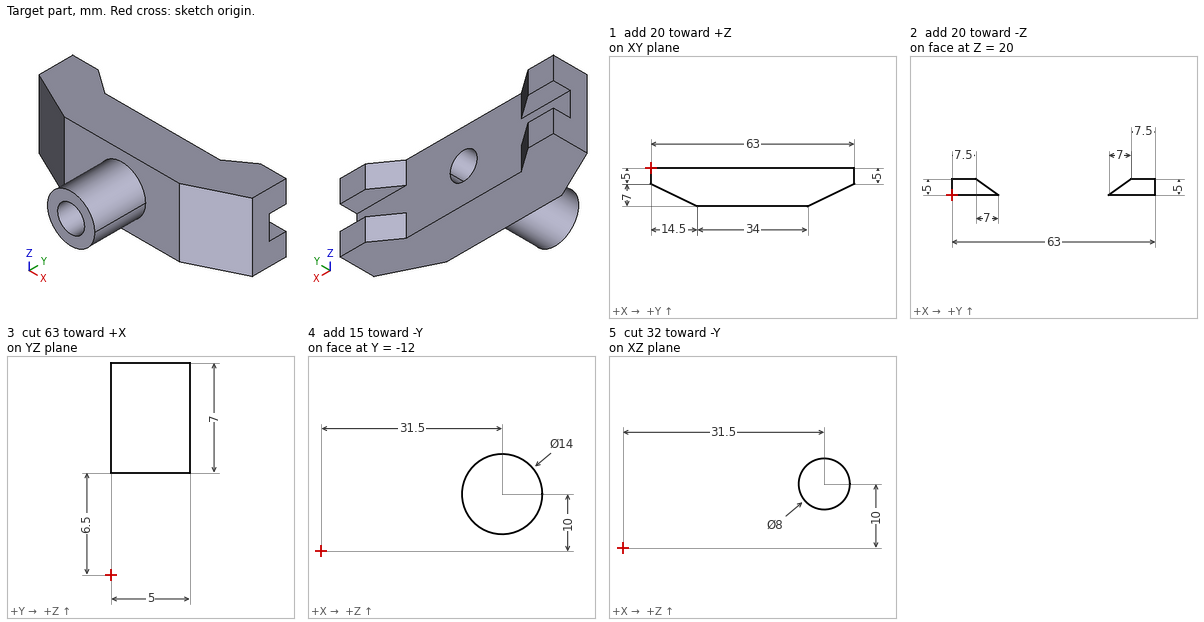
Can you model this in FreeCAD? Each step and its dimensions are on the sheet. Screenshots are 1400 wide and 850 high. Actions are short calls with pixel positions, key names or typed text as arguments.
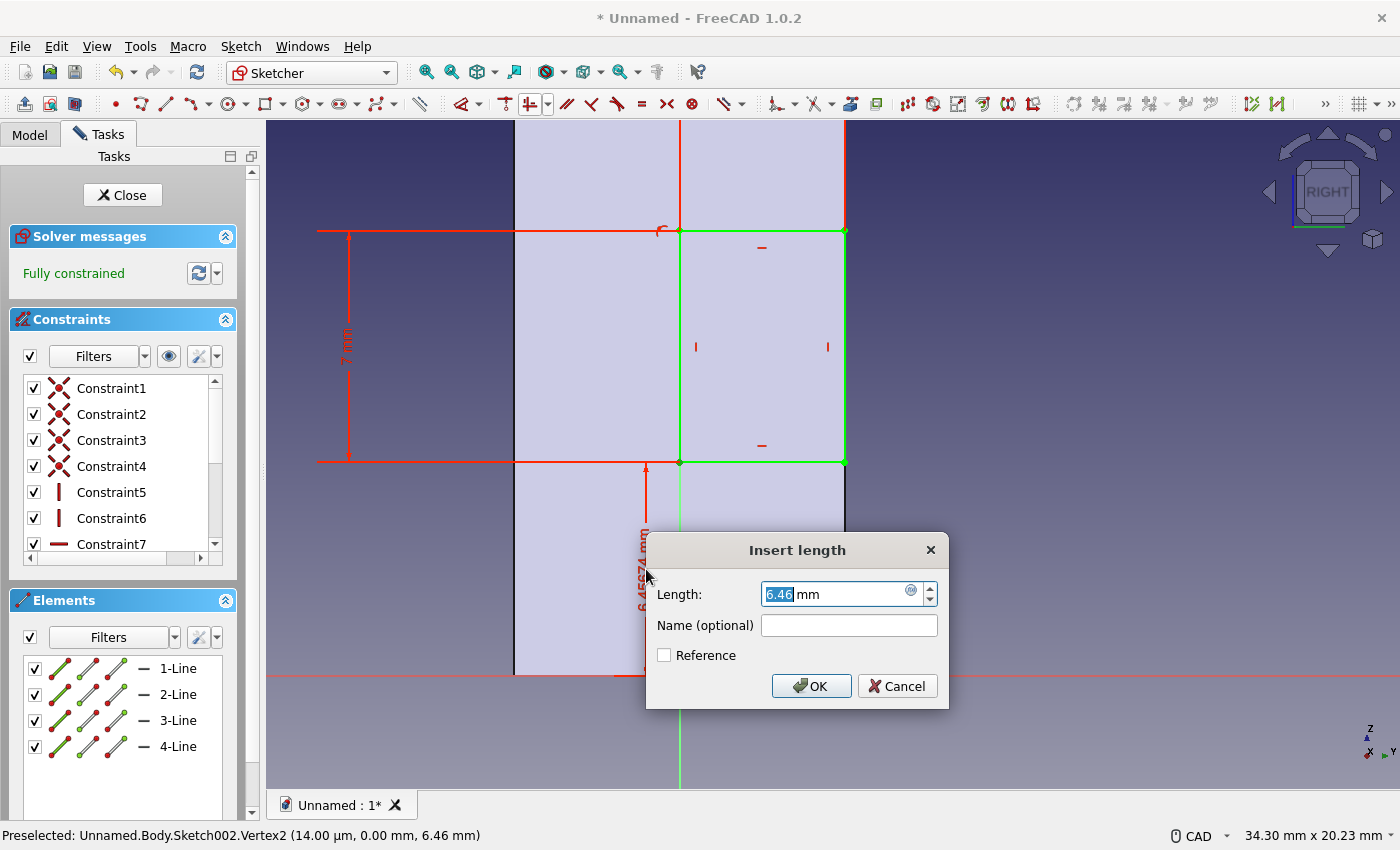
text(6.5)
key(Return)
key(Escape)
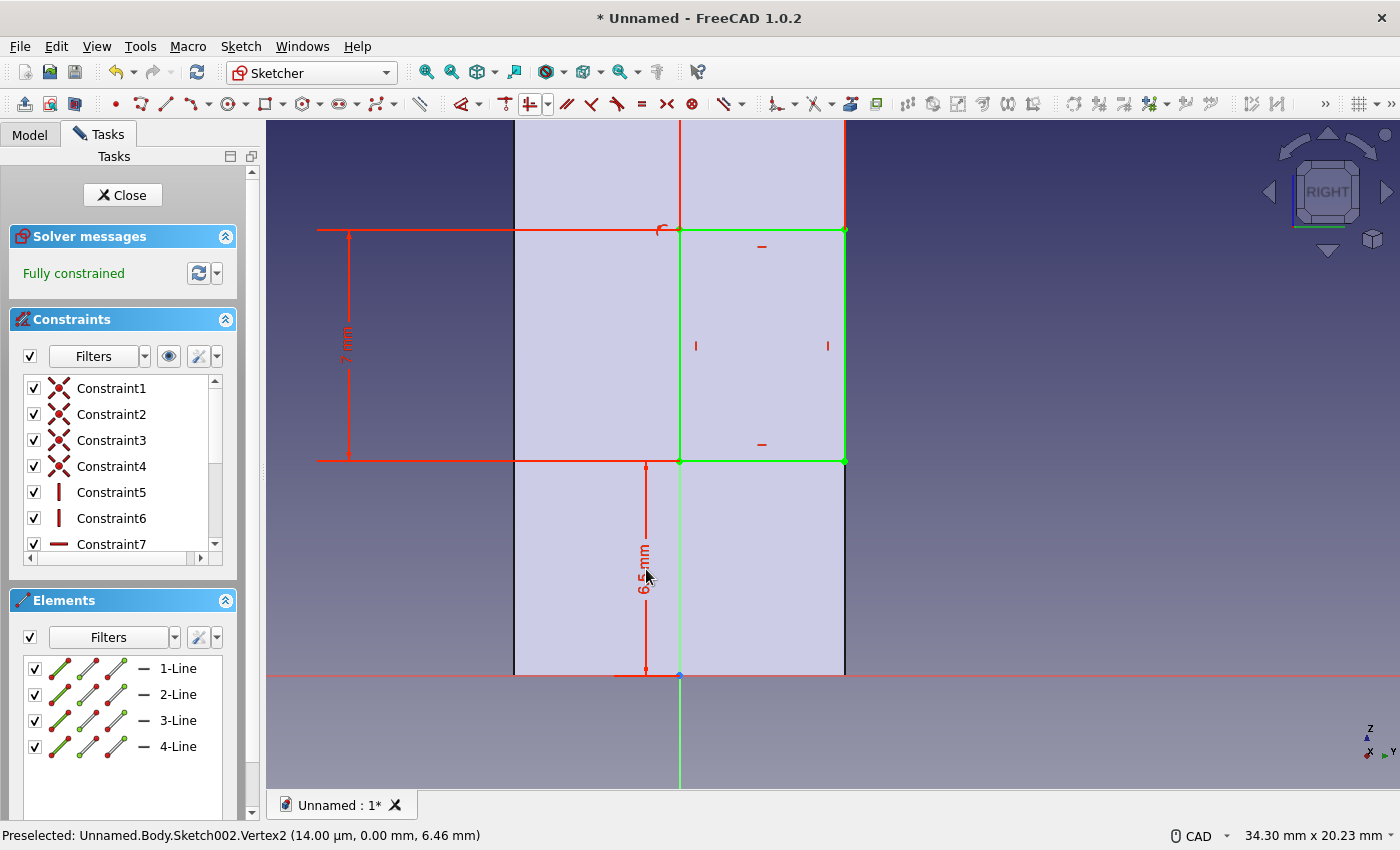
click(123, 195)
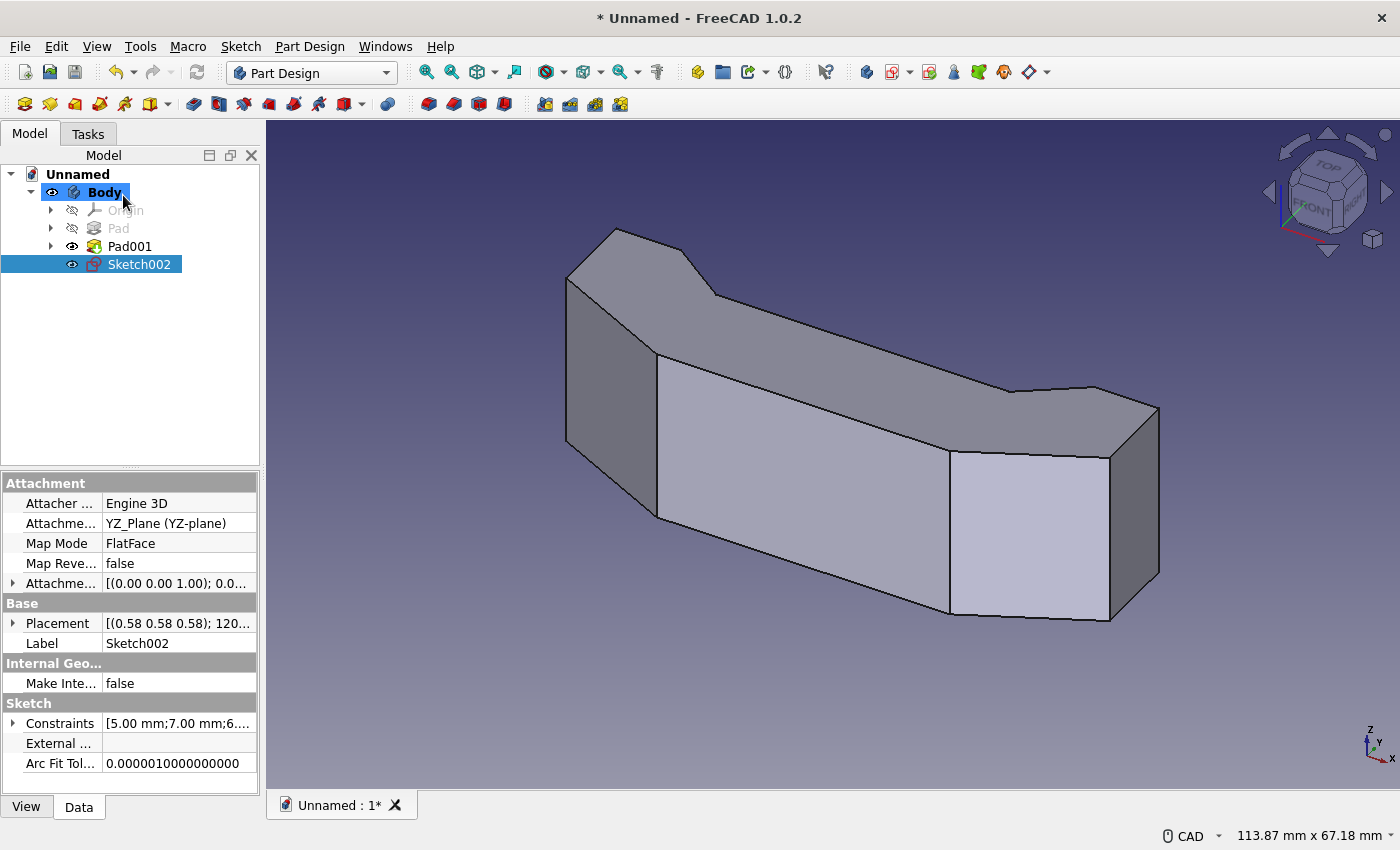
click(194, 104)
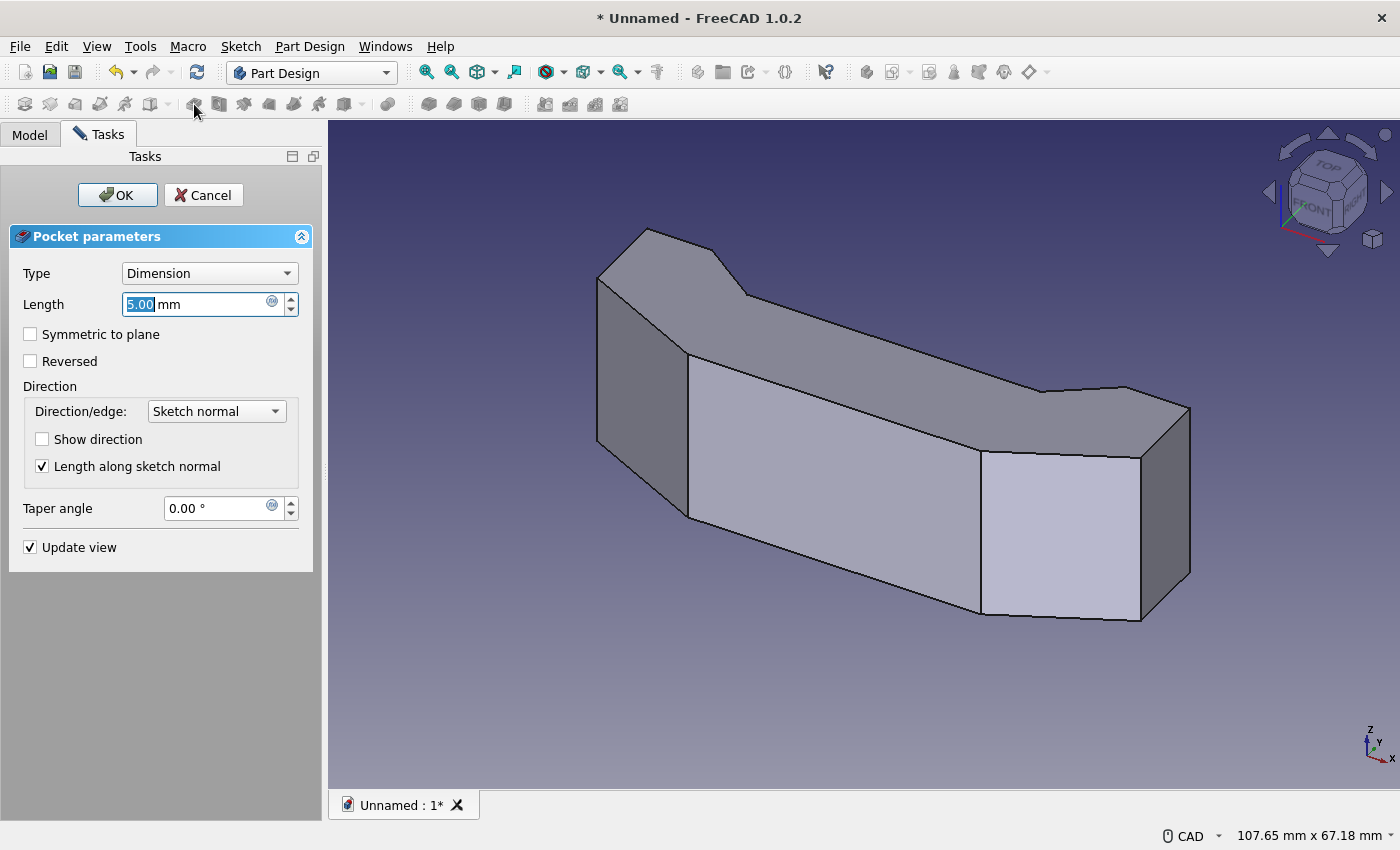
text(63)
key(Tab)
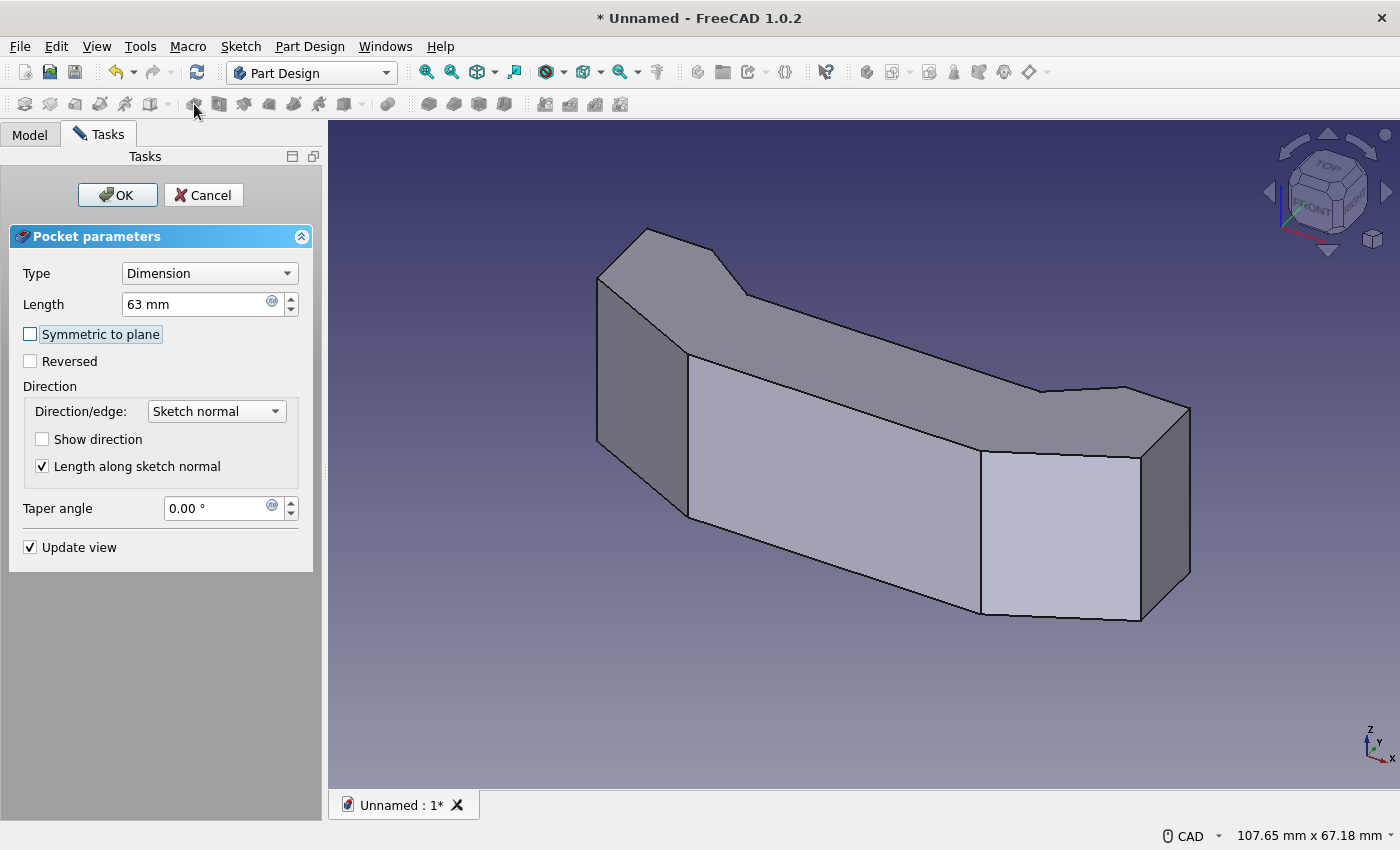
click(31, 361)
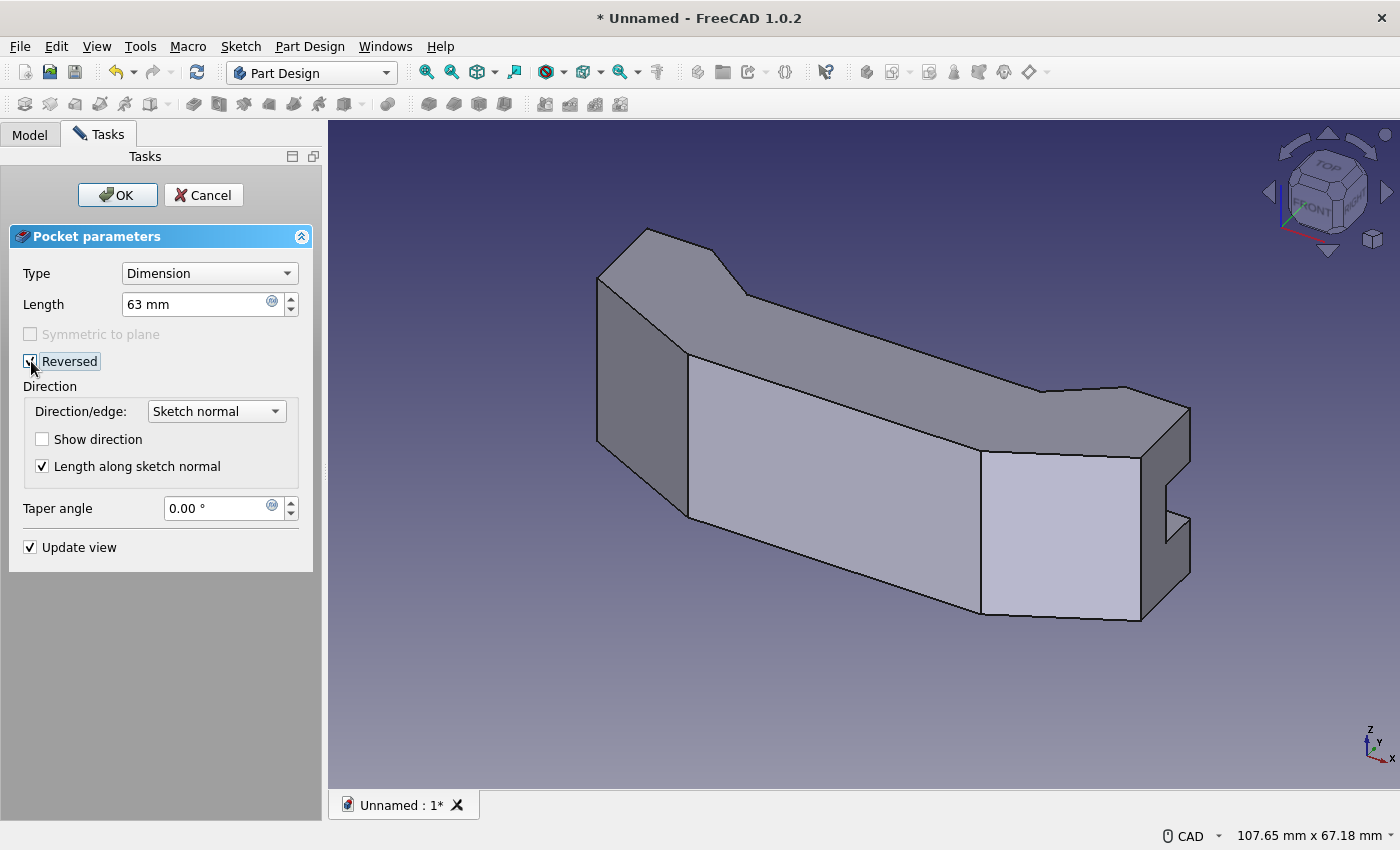
click(118, 195)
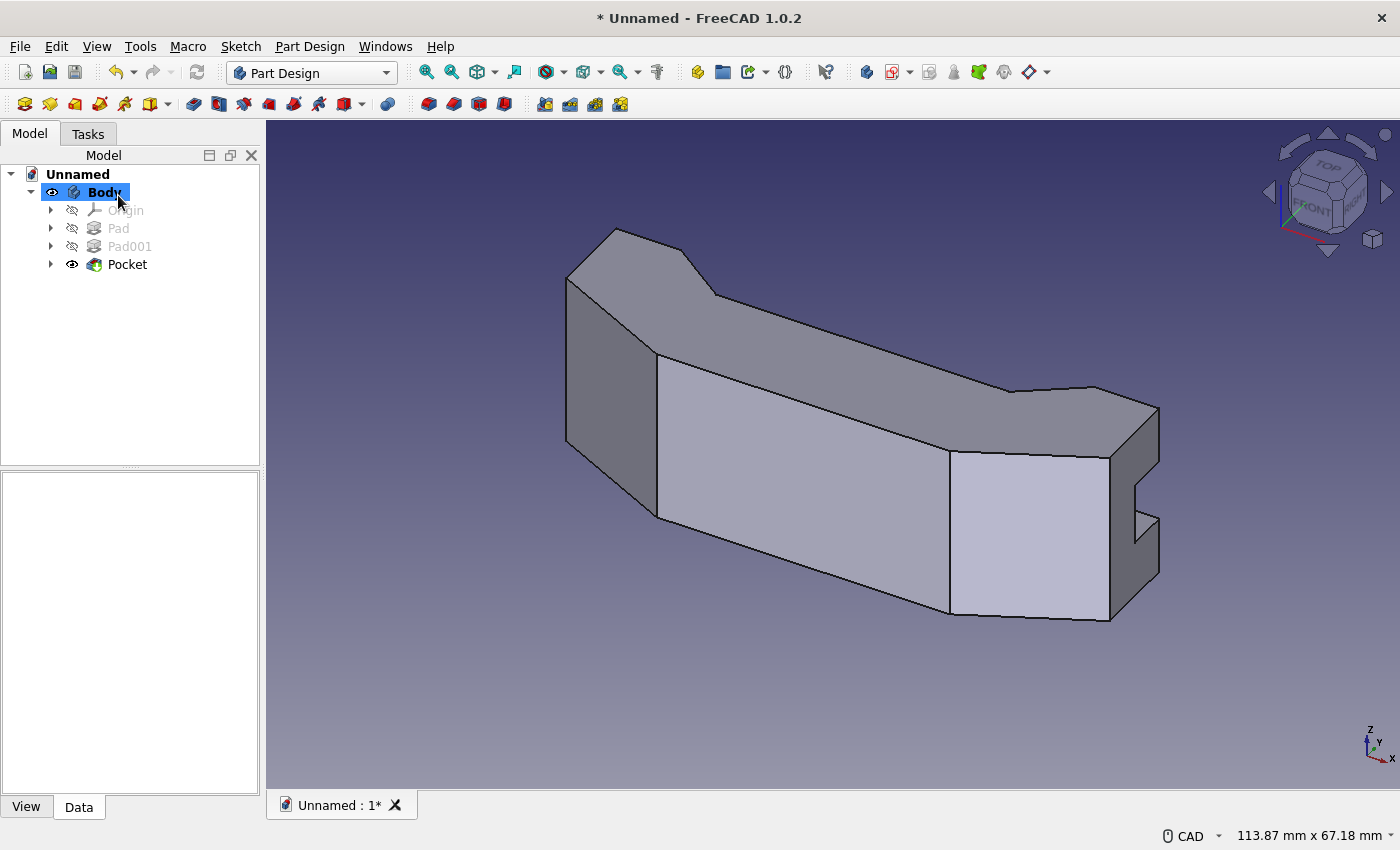
click(845, 497)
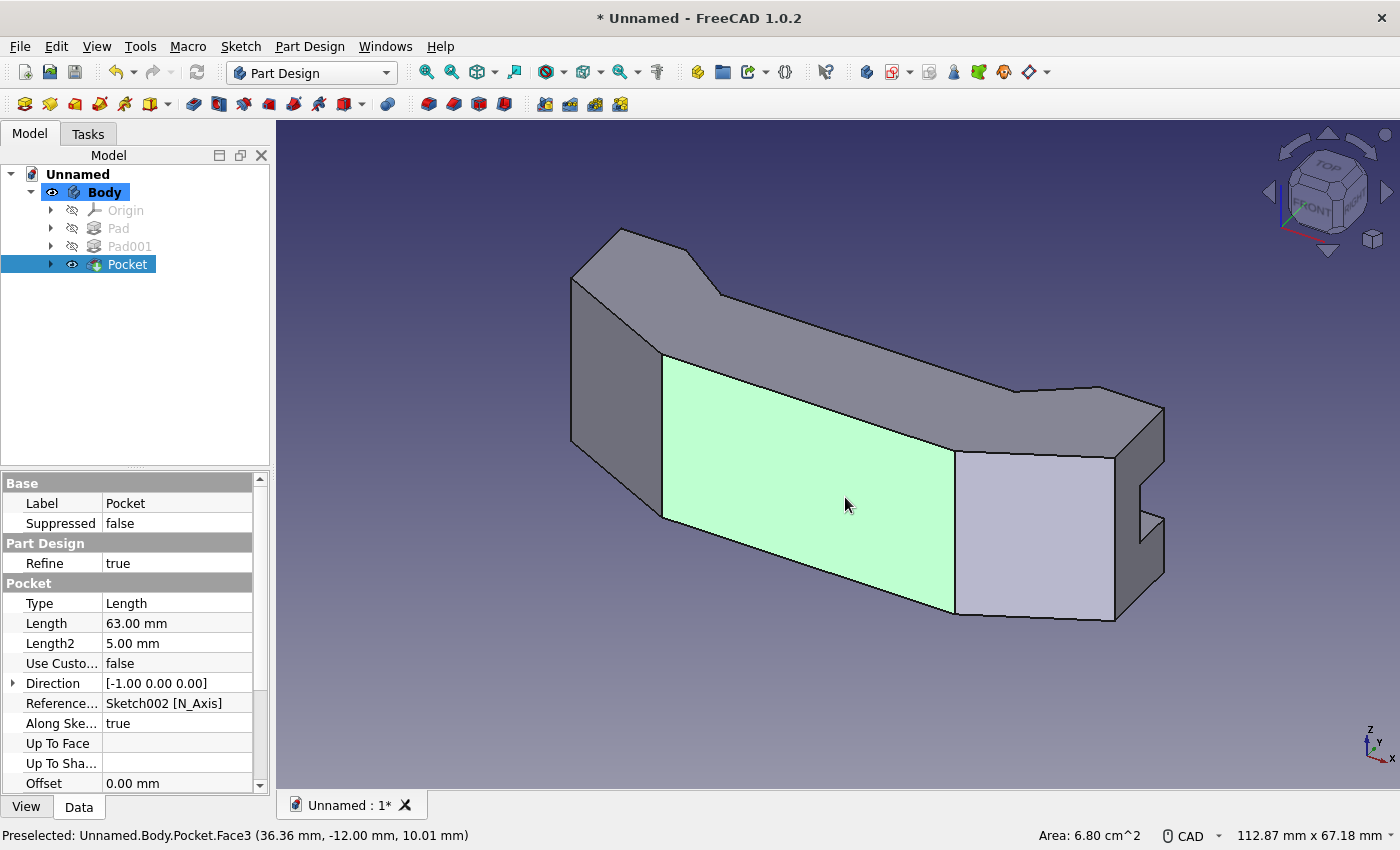
click(892, 72)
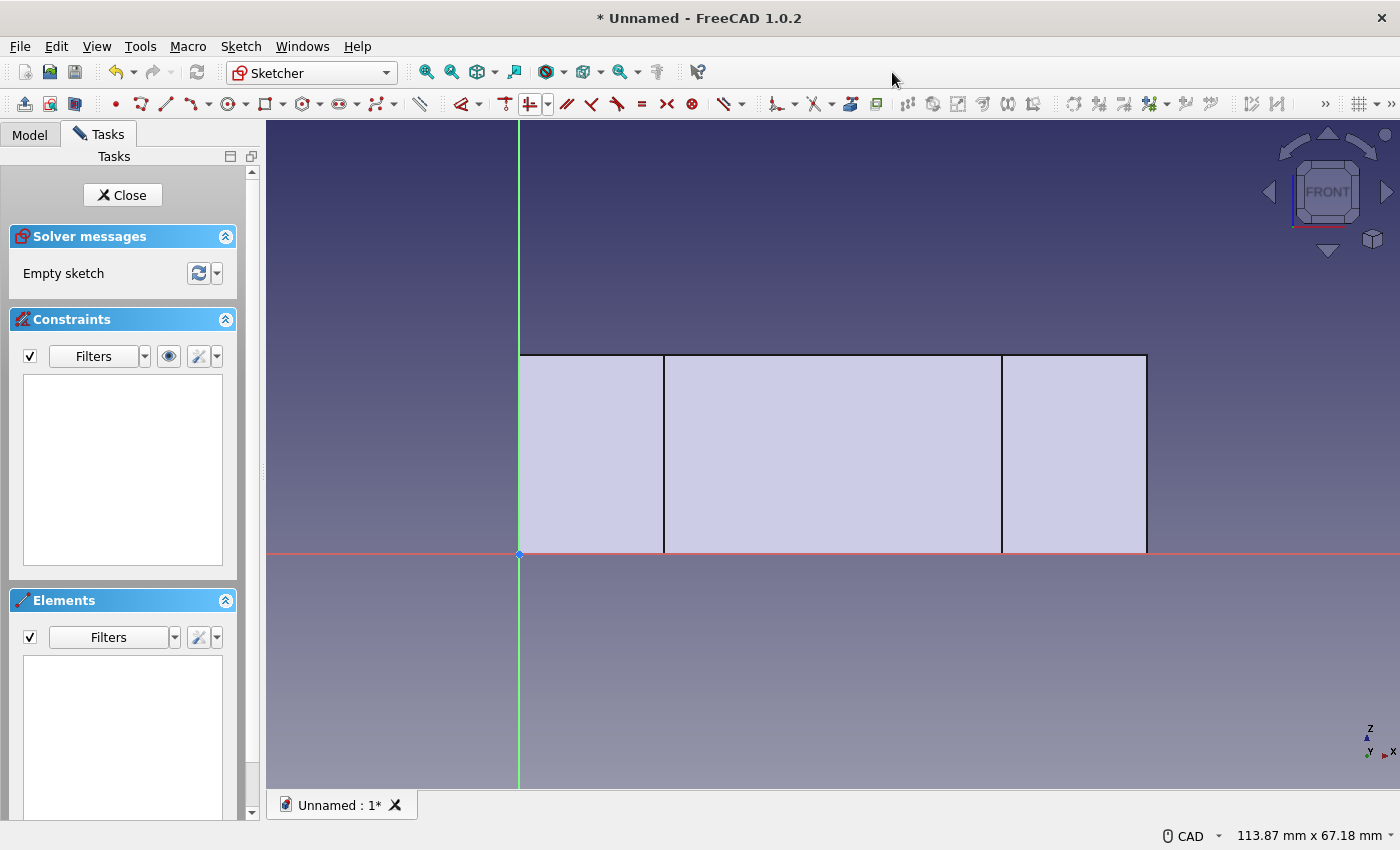
scroll(863, 454, up, 6)